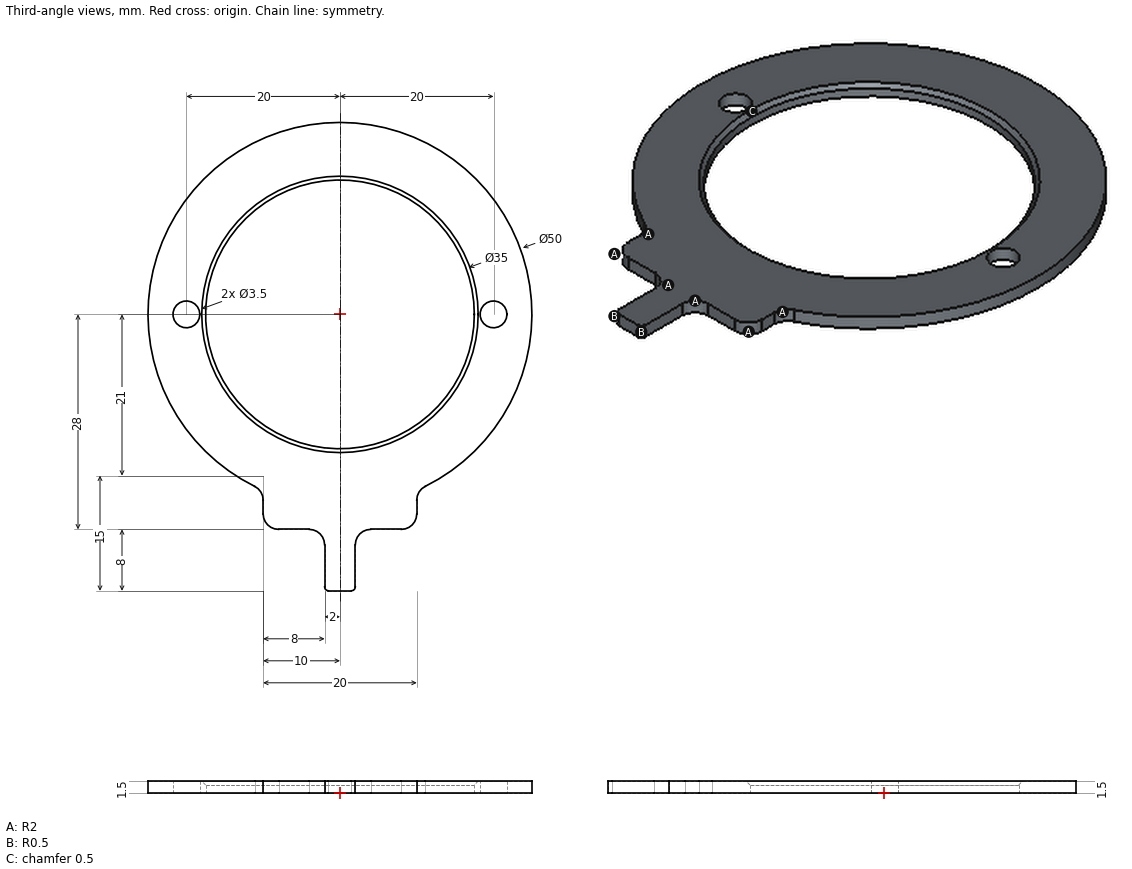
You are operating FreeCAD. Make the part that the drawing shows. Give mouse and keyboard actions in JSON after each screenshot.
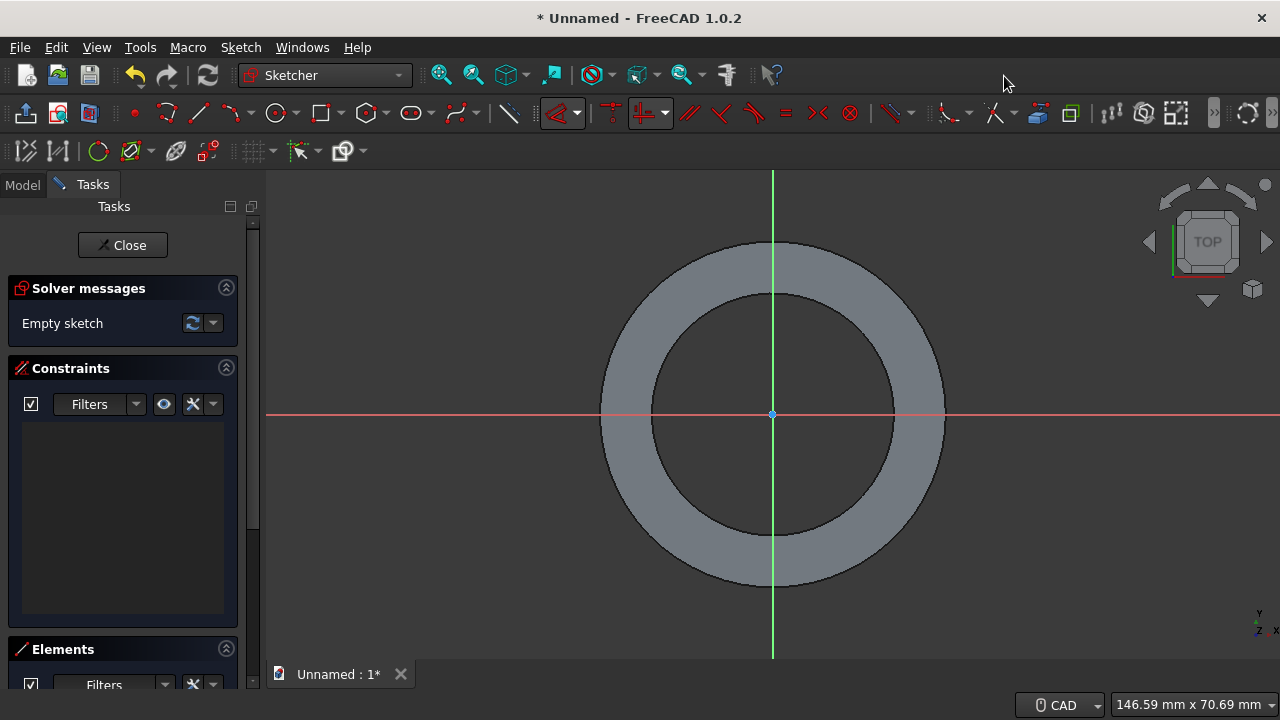
{"action": "scroll", "coordinate": [396, 198], "scroll_direction": "down", "scroll_amount": 1}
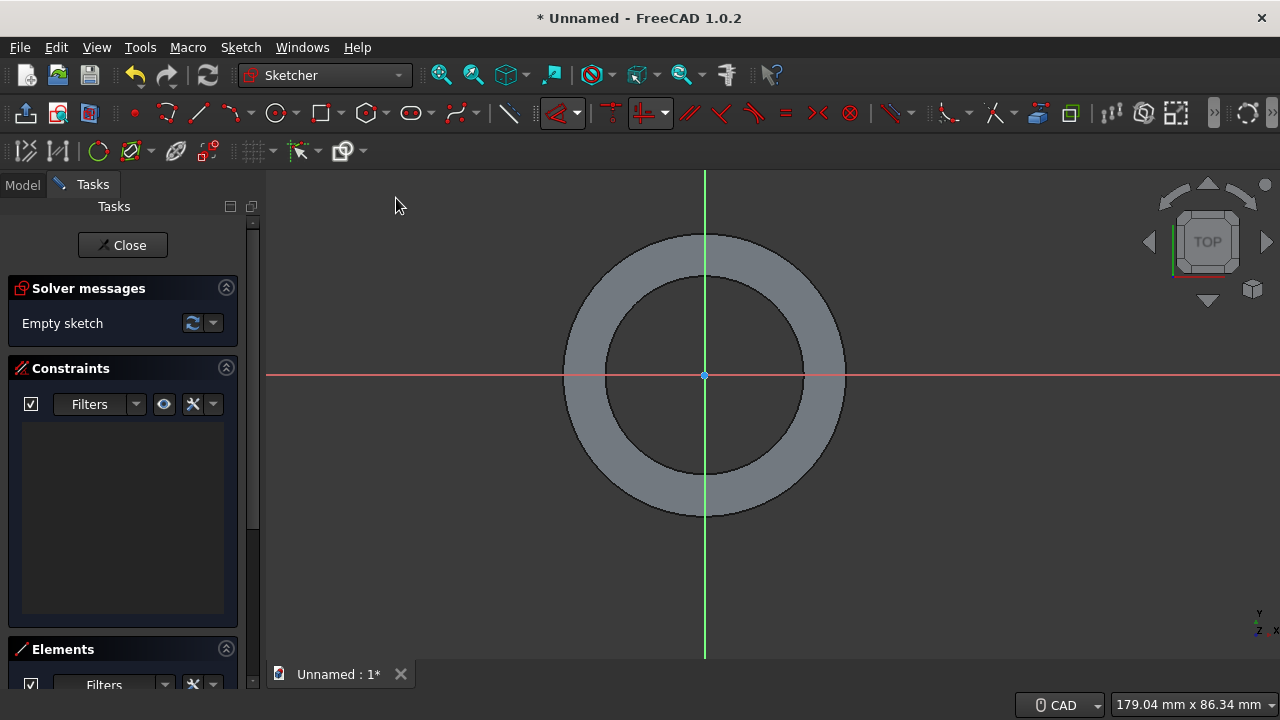
{"action": "scroll", "coordinate": [705, 605], "scroll_direction": "up", "scroll_amount": 2}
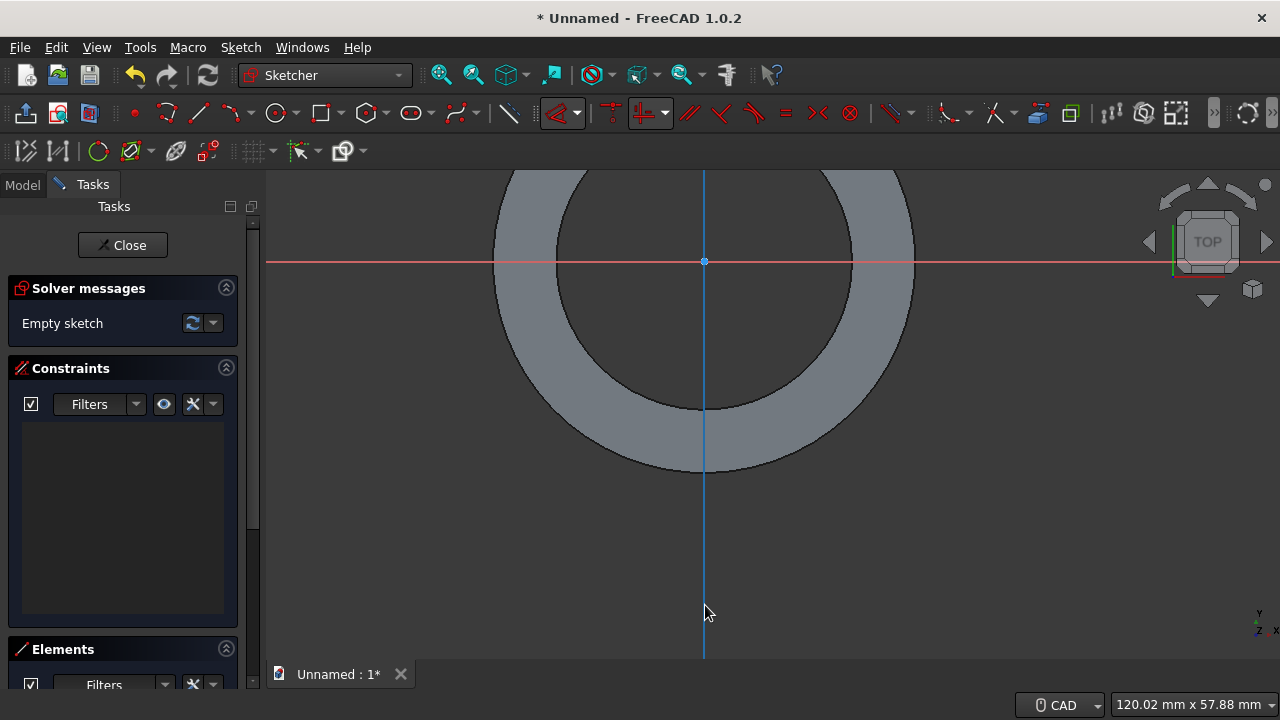
{"action": "left_click", "coordinate": [322, 114]}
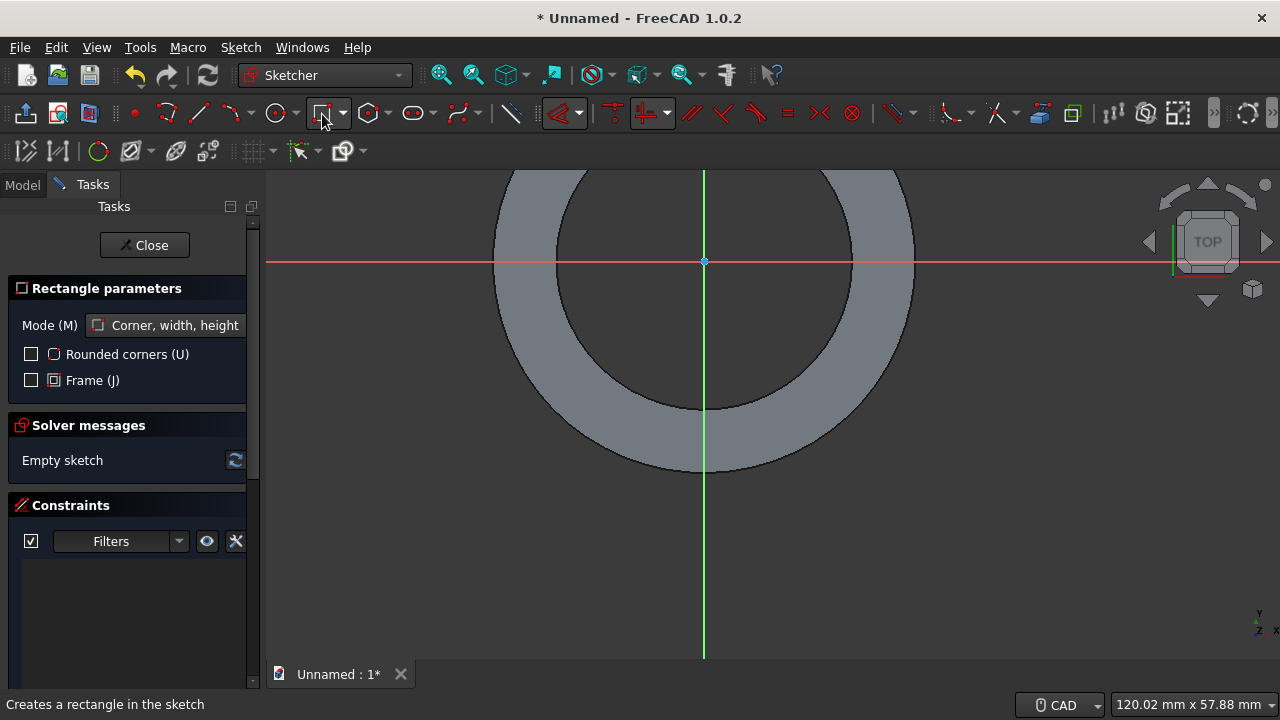
{"action": "left_click", "coordinate": [620, 439]}
{"action": "left_click", "coordinate": [789, 566]}
{"action": "key", "text": "Escape"}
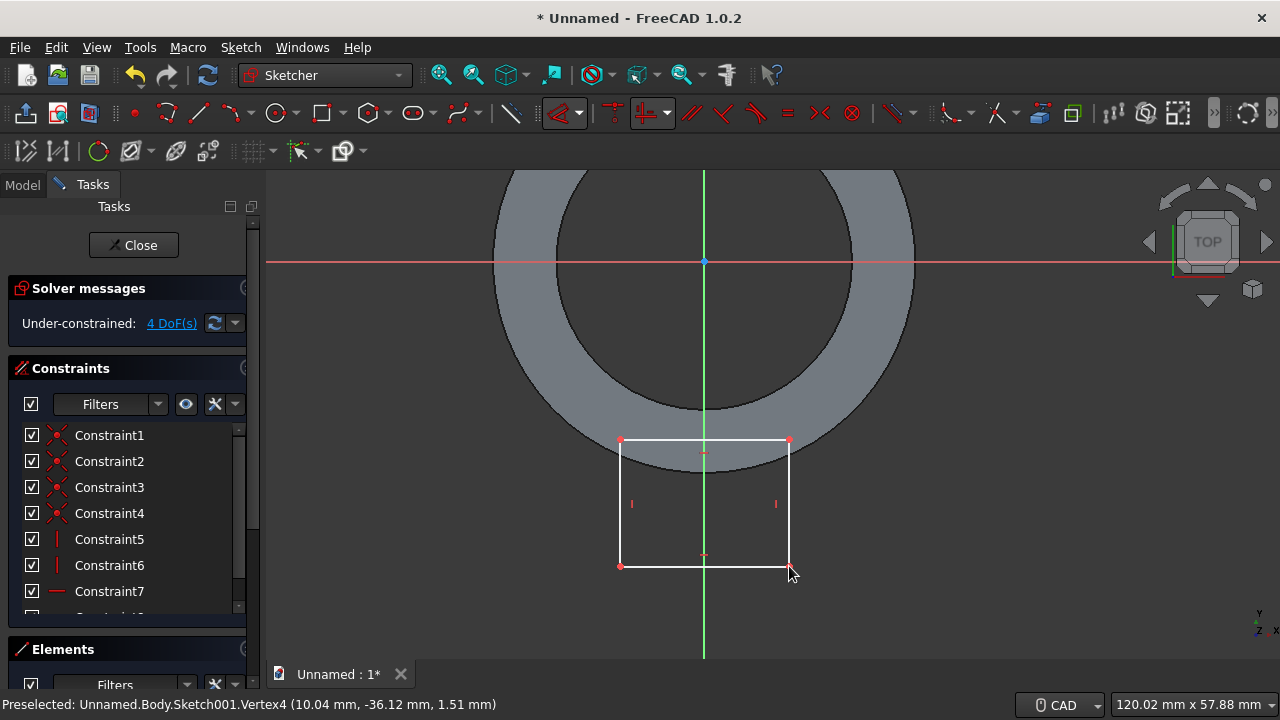
{"action": "left_click", "coordinate": [620, 478]}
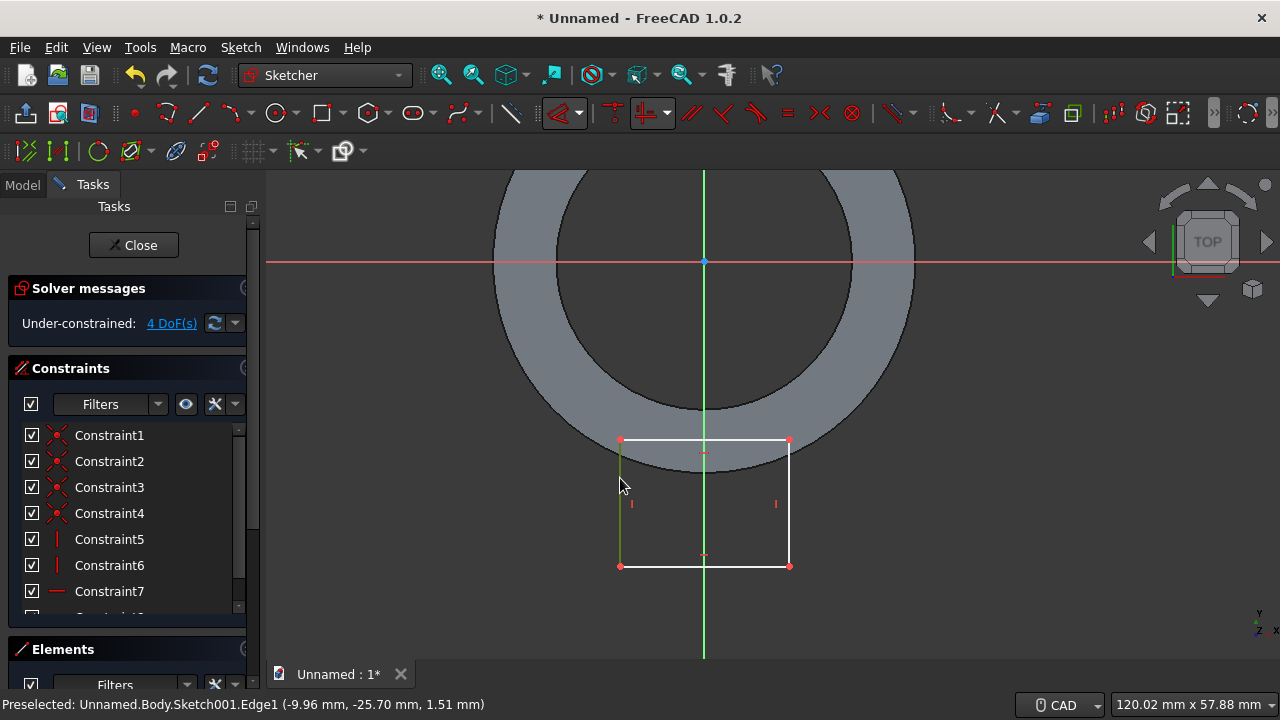
{"action": "left_click", "coordinate": [582, 114]}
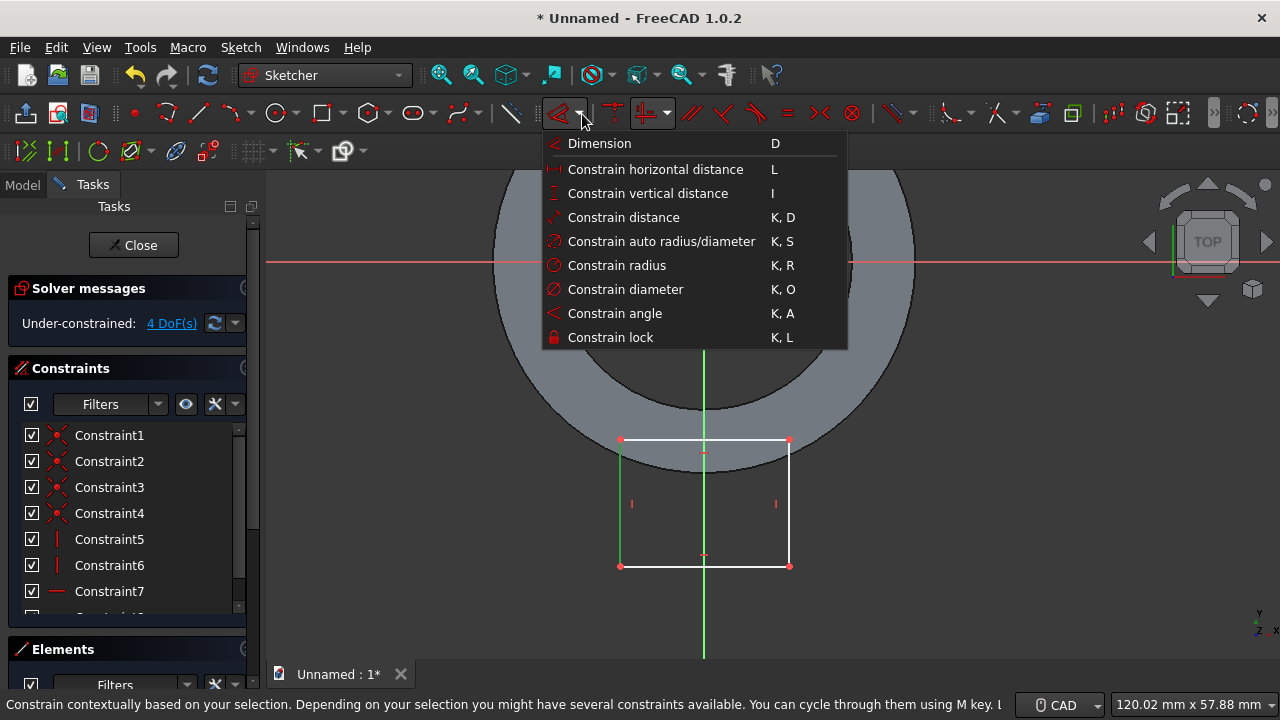
{"action": "left_click", "coordinate": [695, 193]}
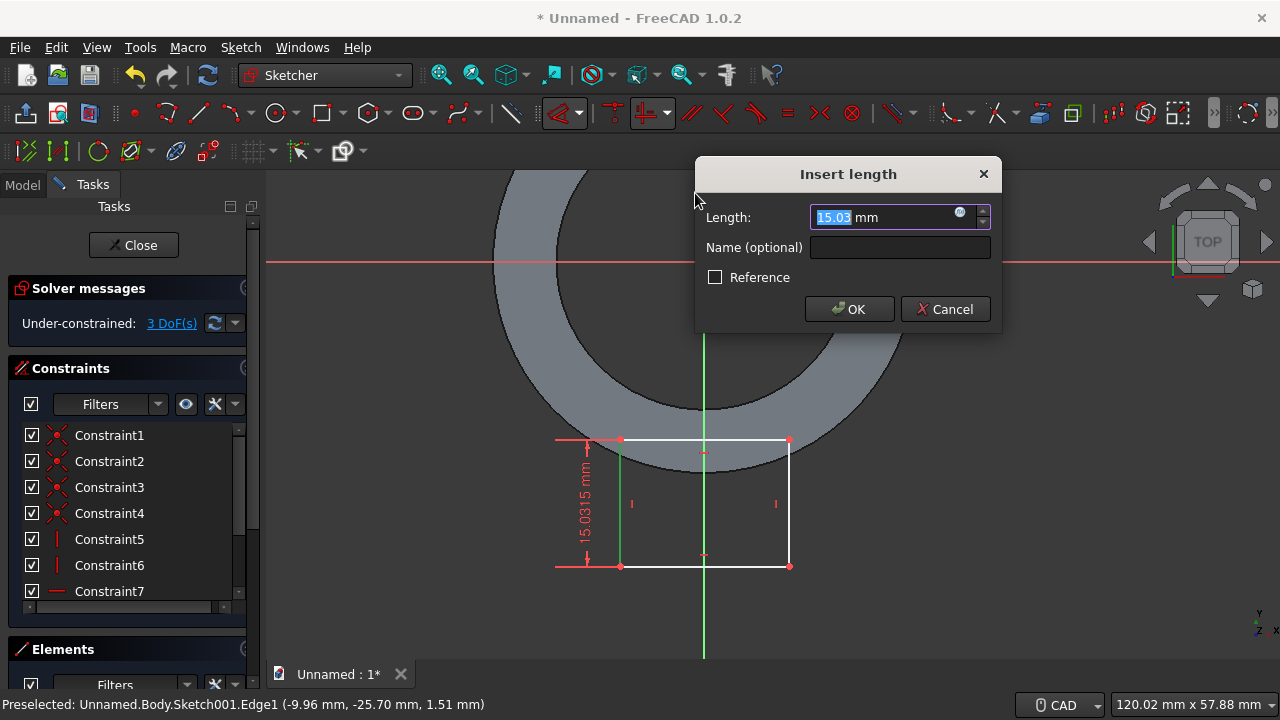
{"action": "type", "text": "15"}
{"action": "key", "text": "Return"}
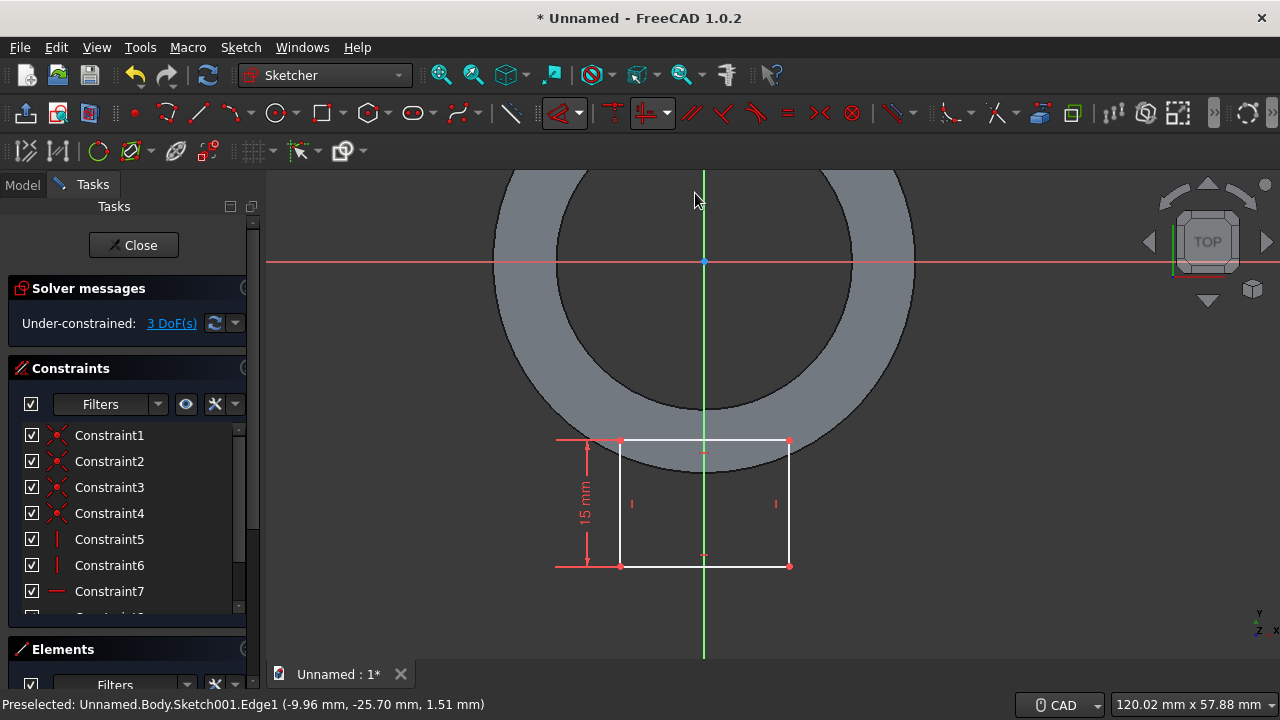
{"action": "left_click", "coordinate": [671, 567]}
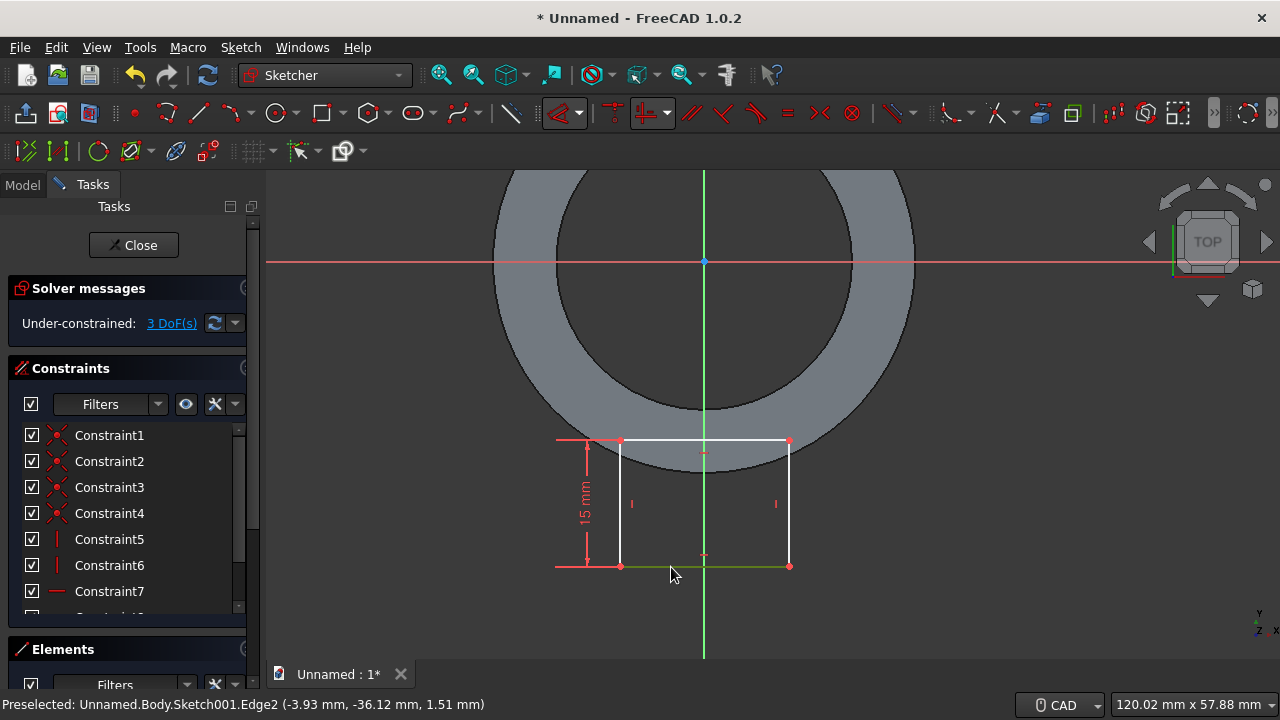
{"action": "key", "text": "l"}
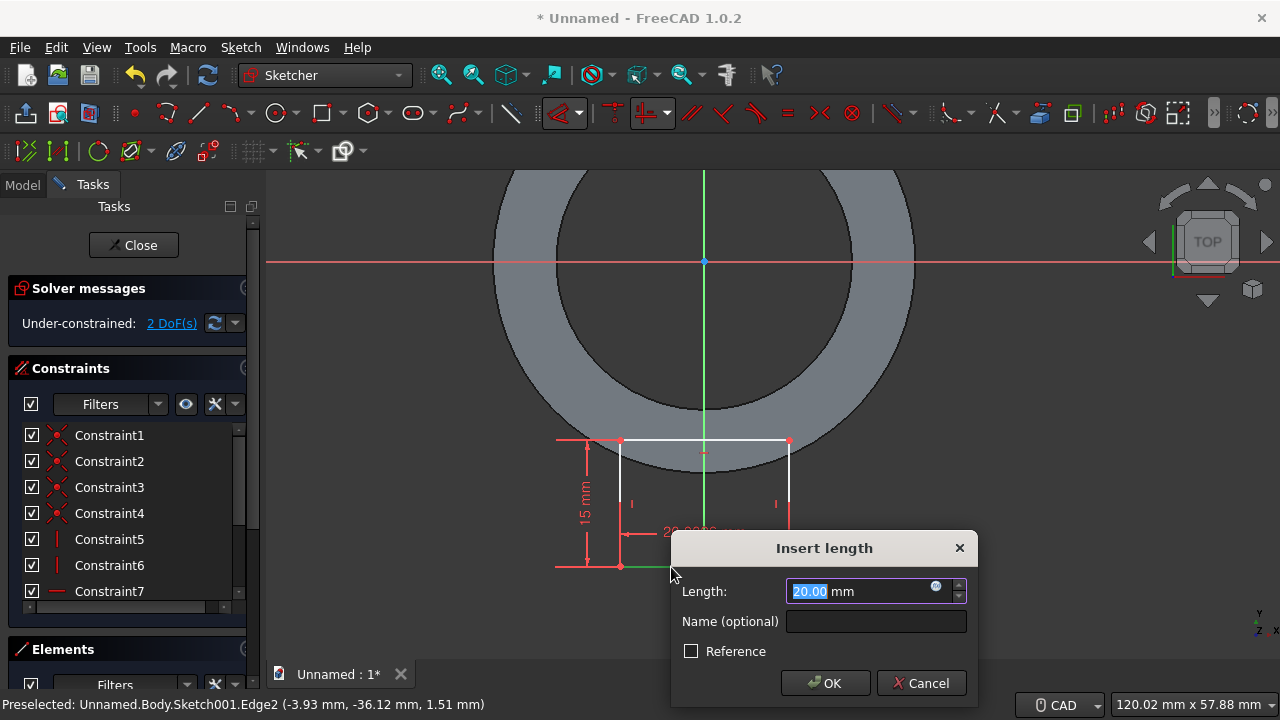
{"action": "type", "text": "20"}
{"action": "key", "text": "Return"}